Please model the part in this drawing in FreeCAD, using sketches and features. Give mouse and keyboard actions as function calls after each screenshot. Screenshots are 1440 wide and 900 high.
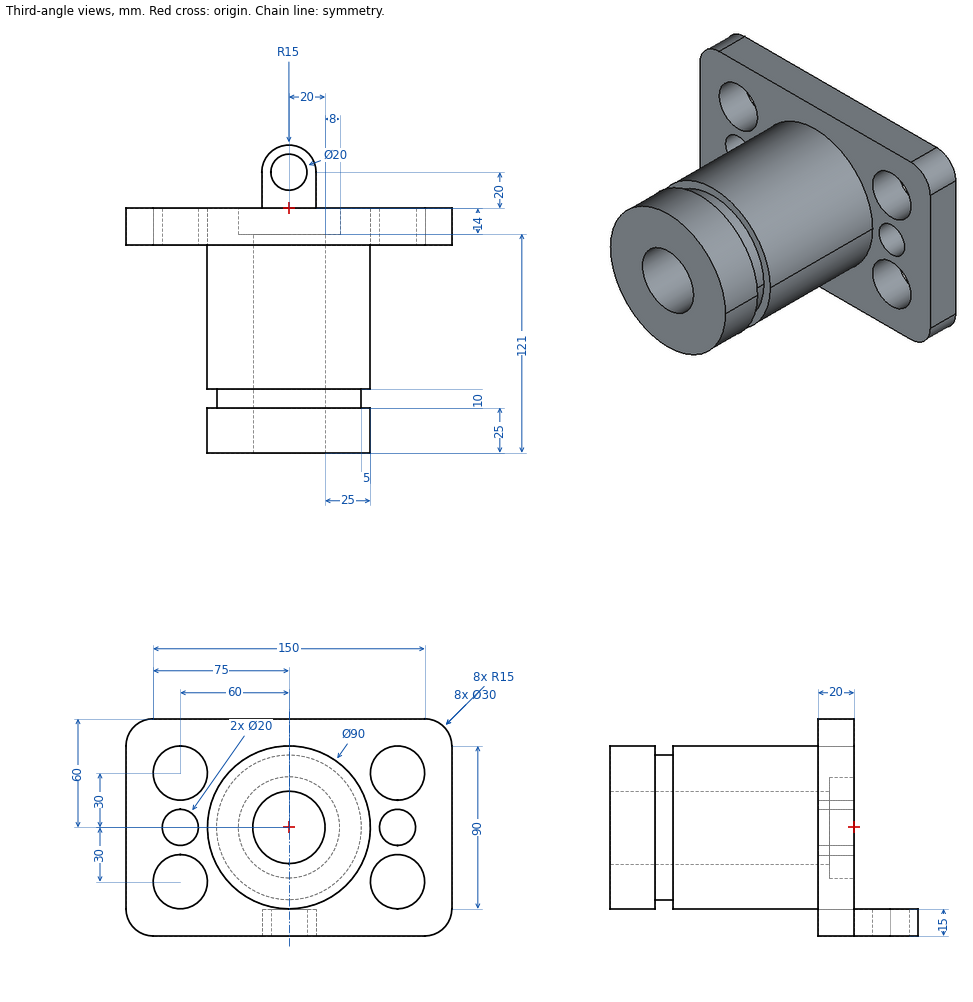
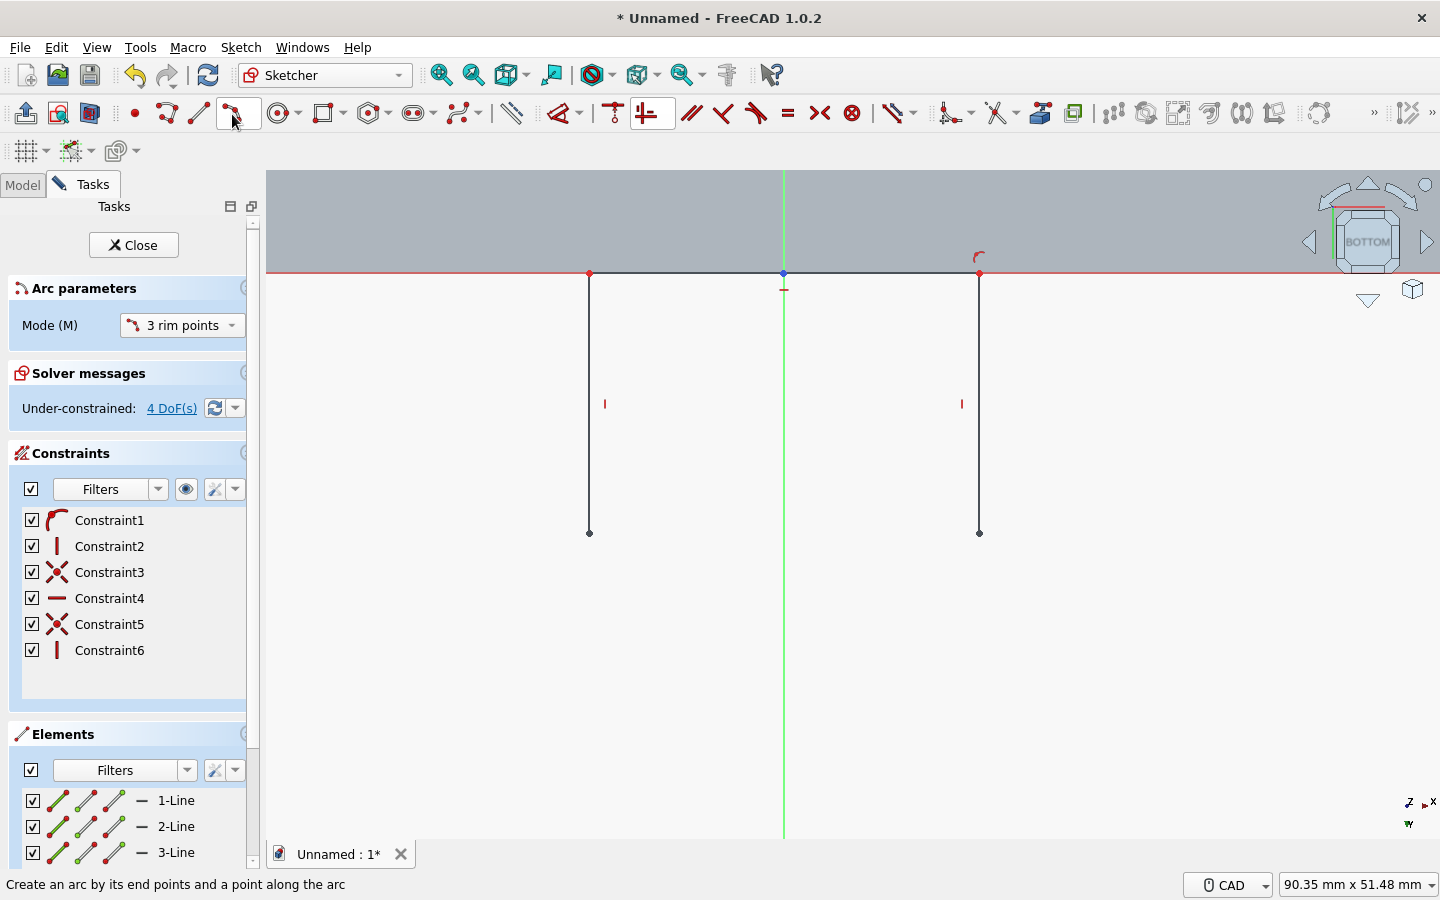
click(589, 534)
click(979, 534)
click(724, 718)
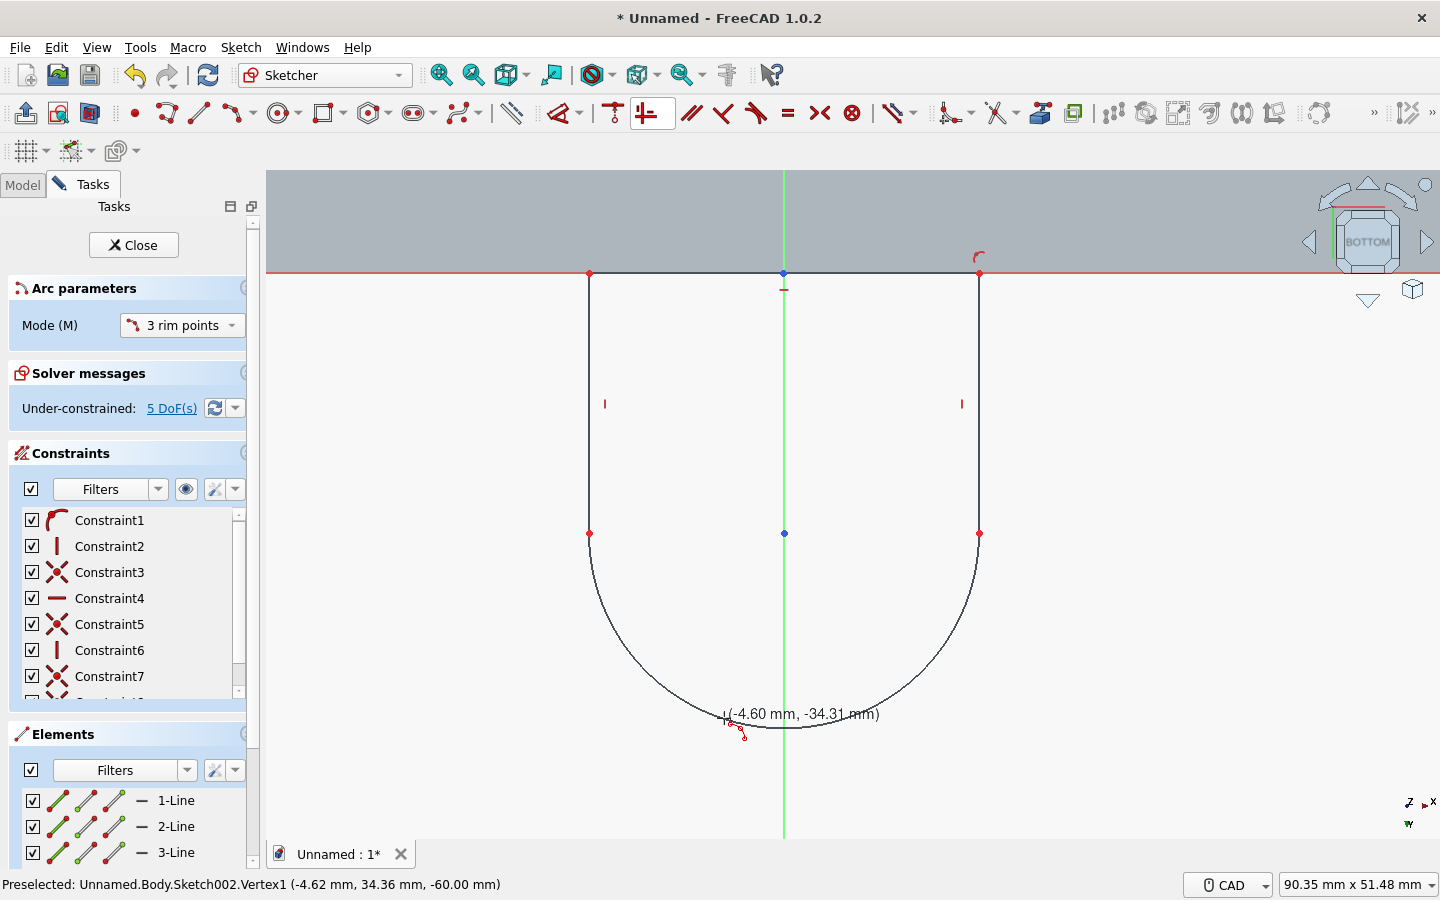
click(278, 114)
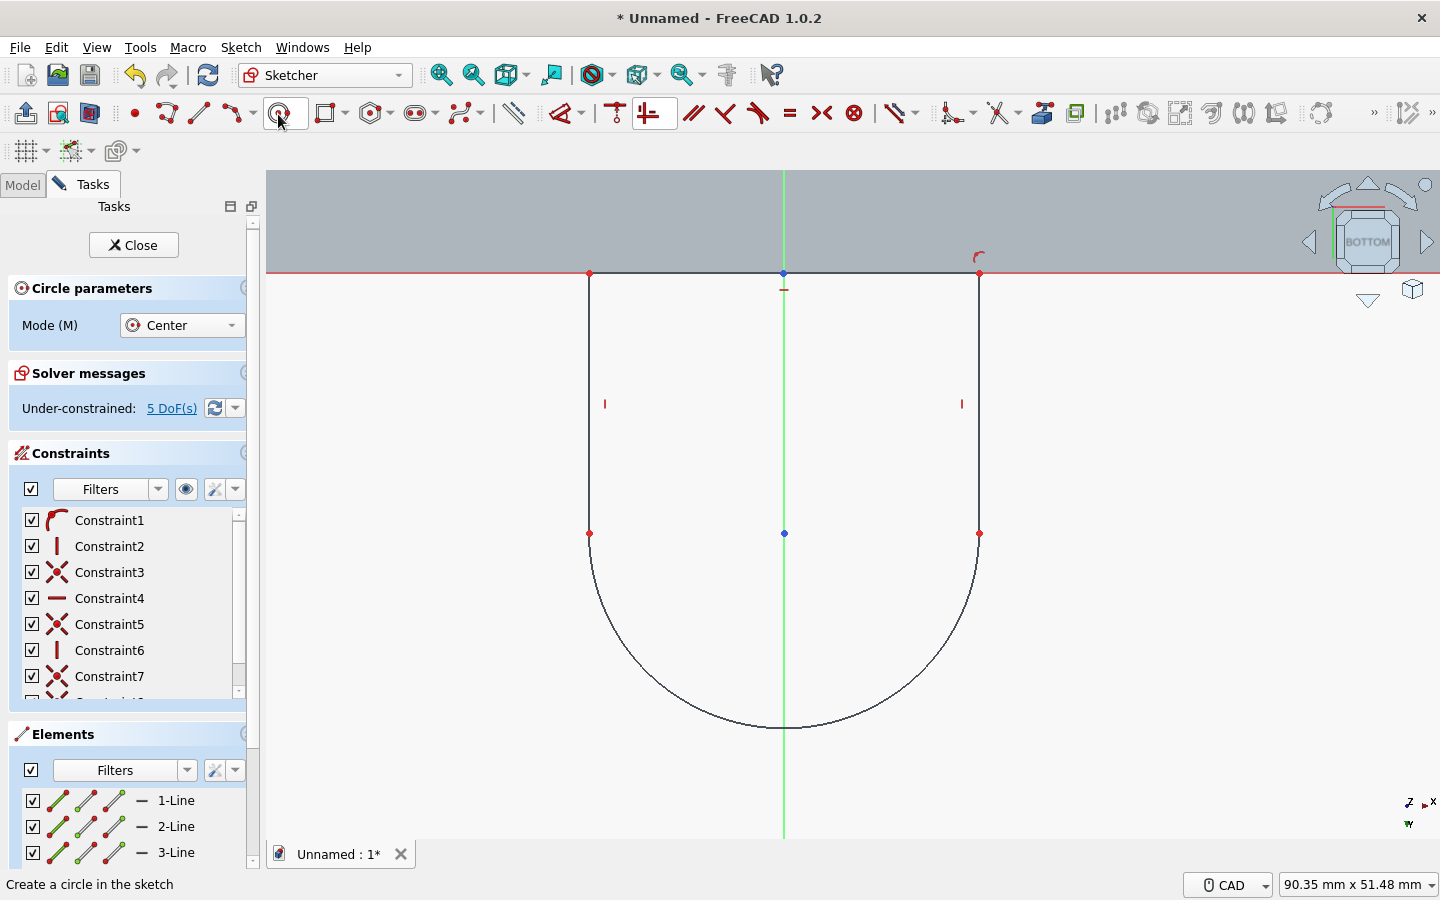
click(784, 533)
move(876, 441)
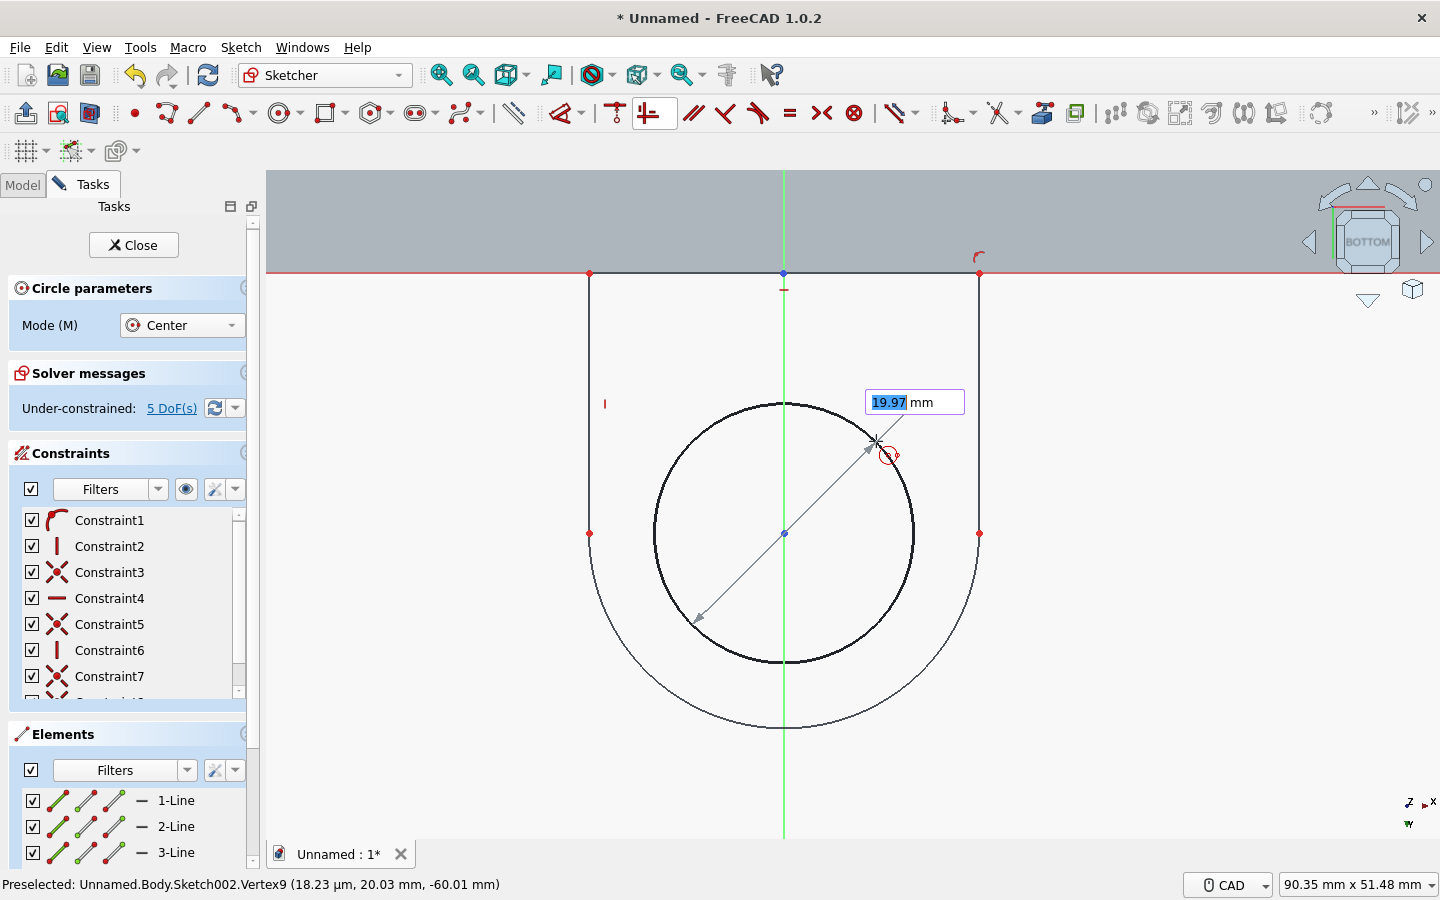
text(20)
key(Return)
key(Escape)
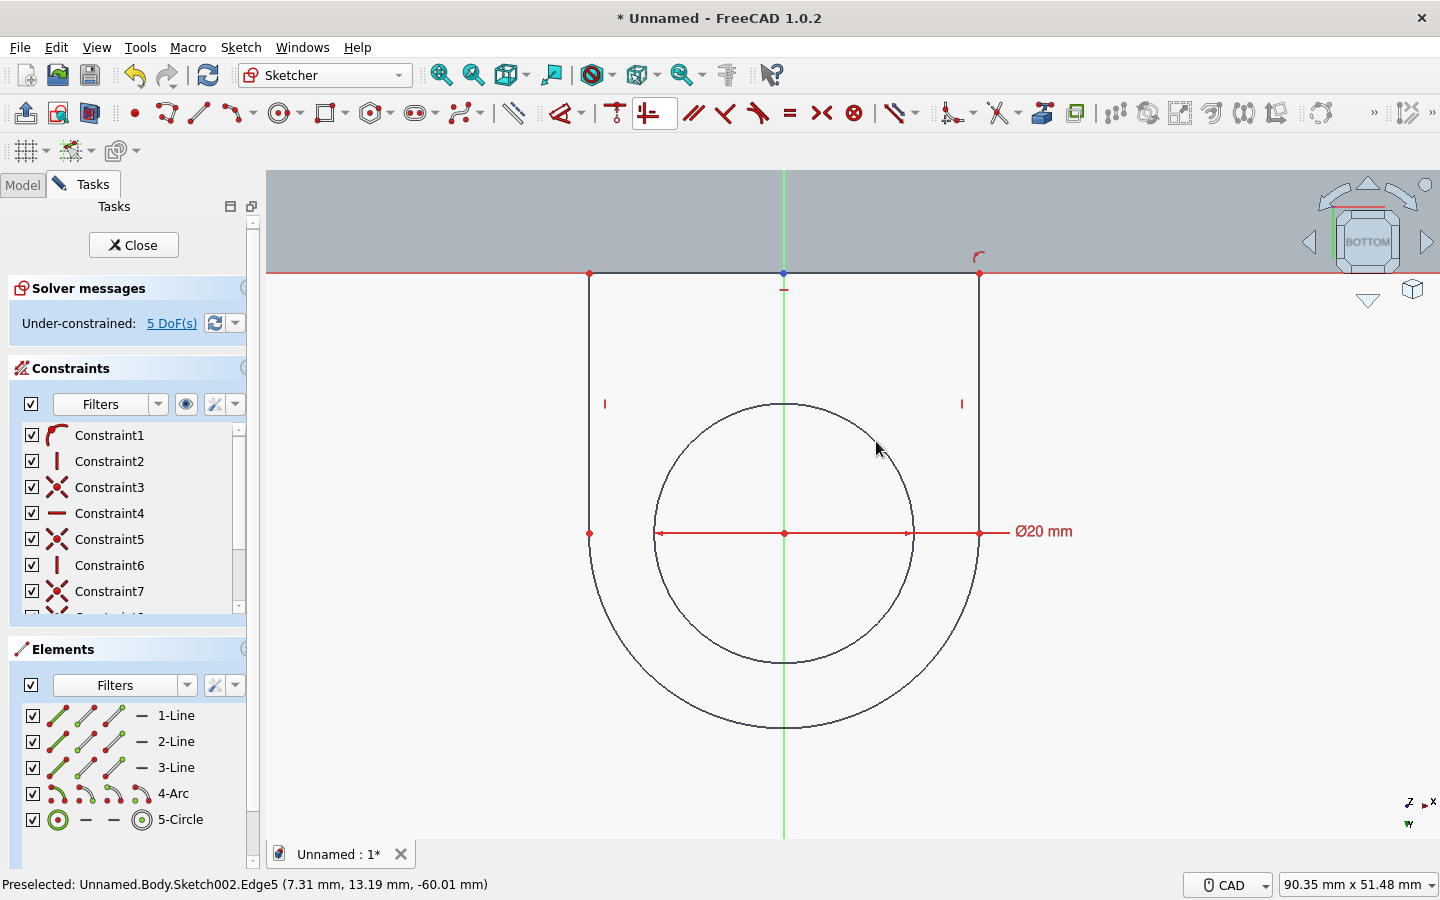
click(979, 456)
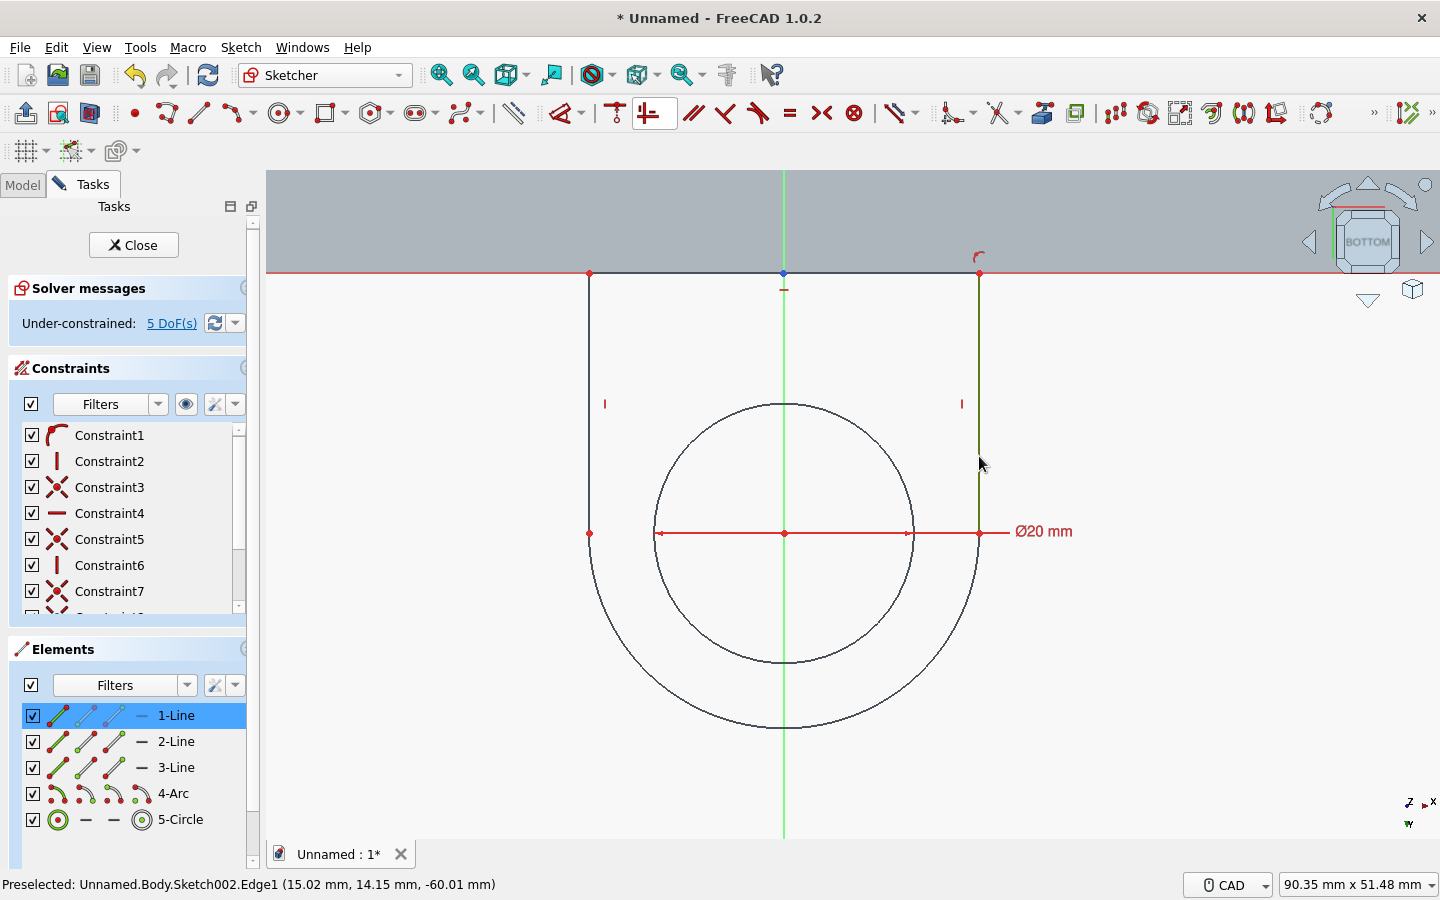
click(670, 691)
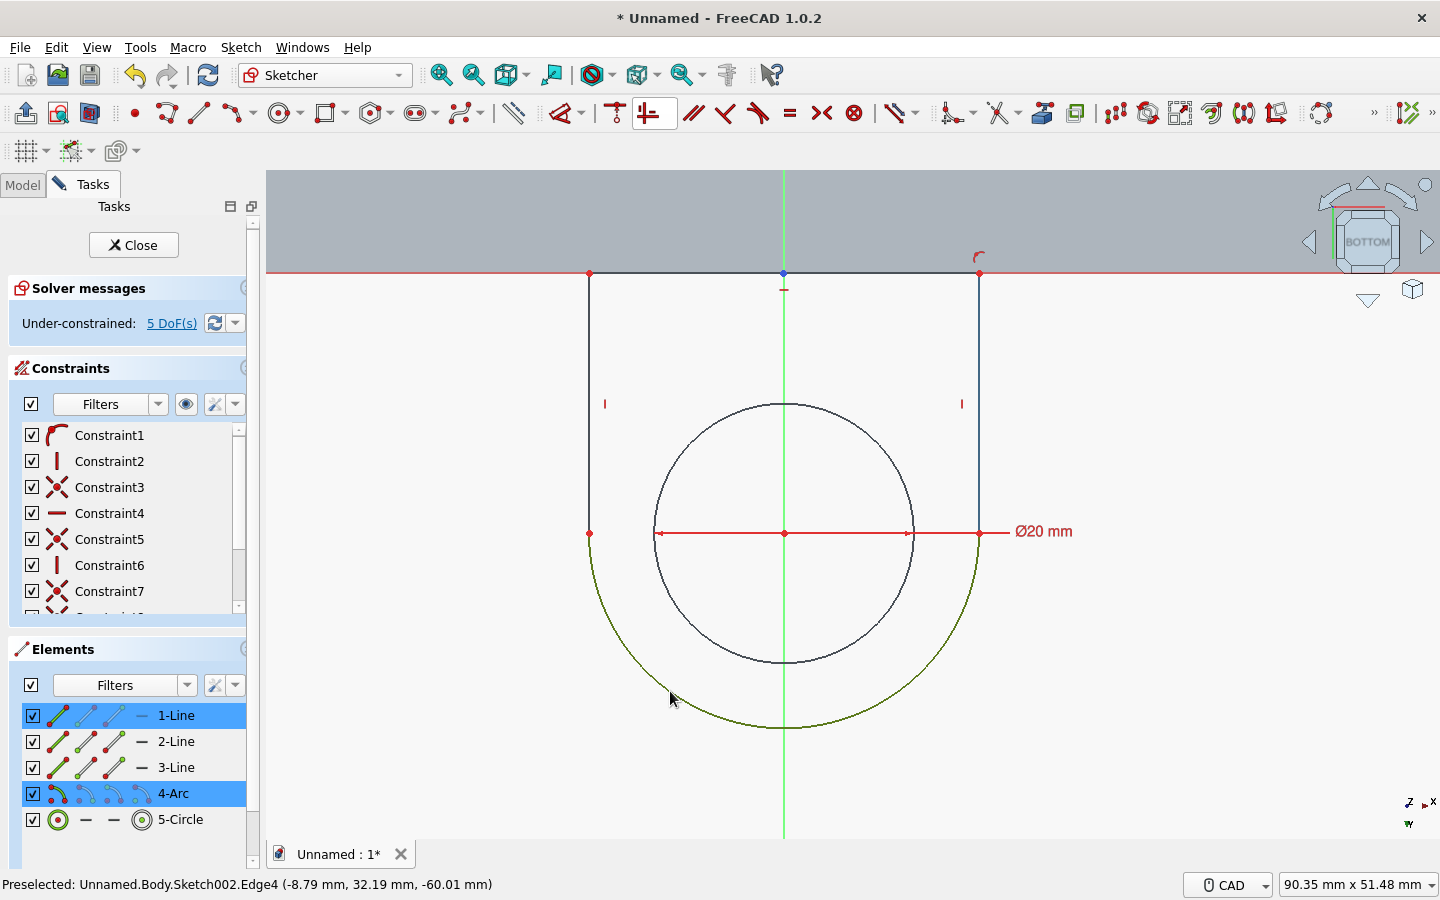
click(758, 114)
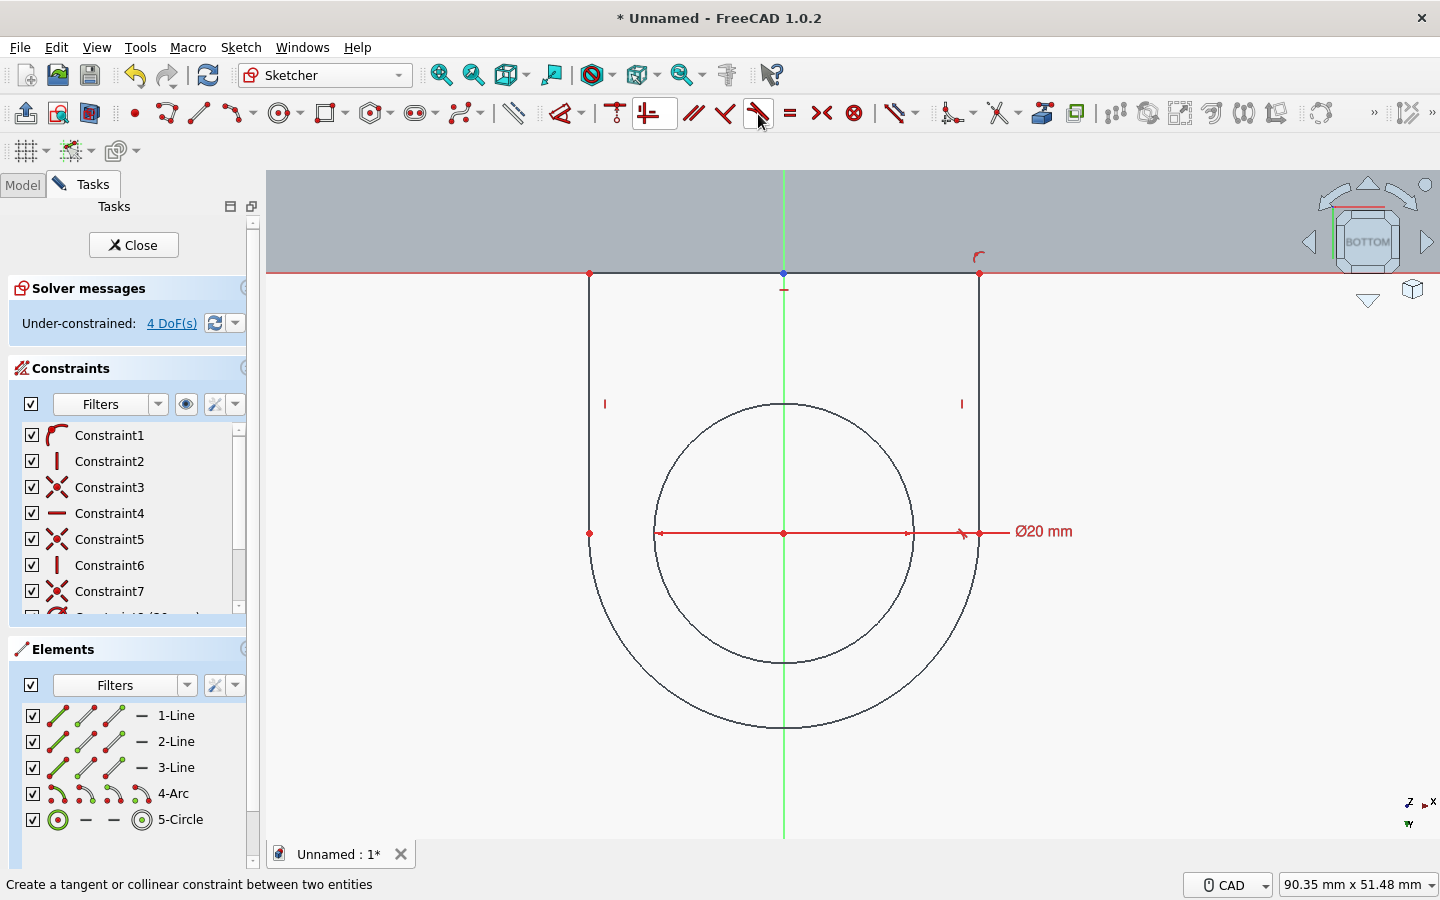
click(589, 351)